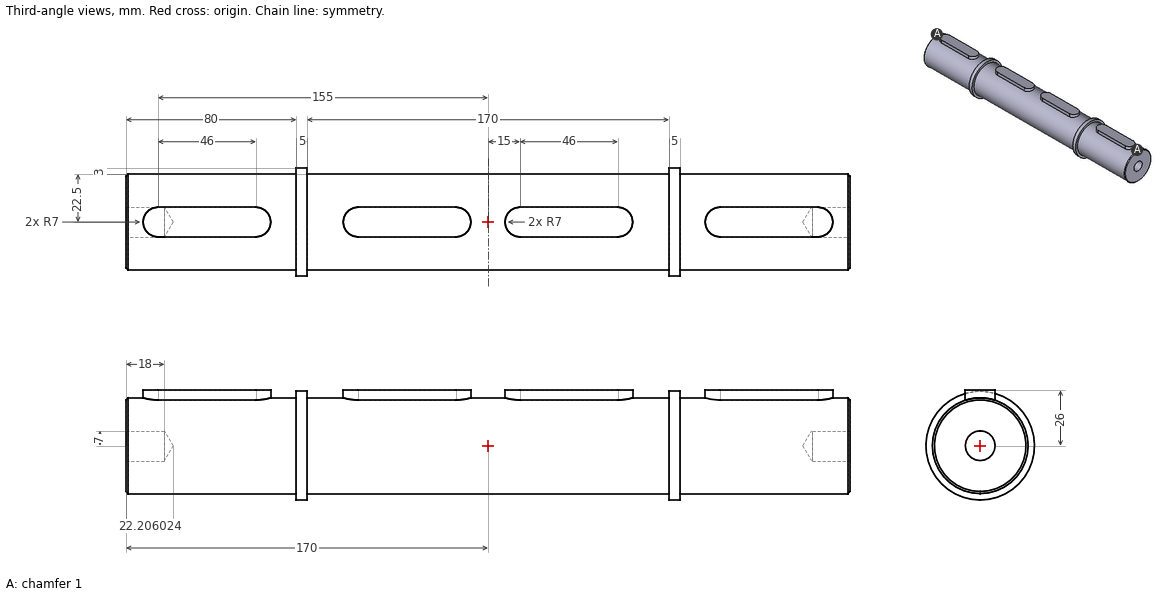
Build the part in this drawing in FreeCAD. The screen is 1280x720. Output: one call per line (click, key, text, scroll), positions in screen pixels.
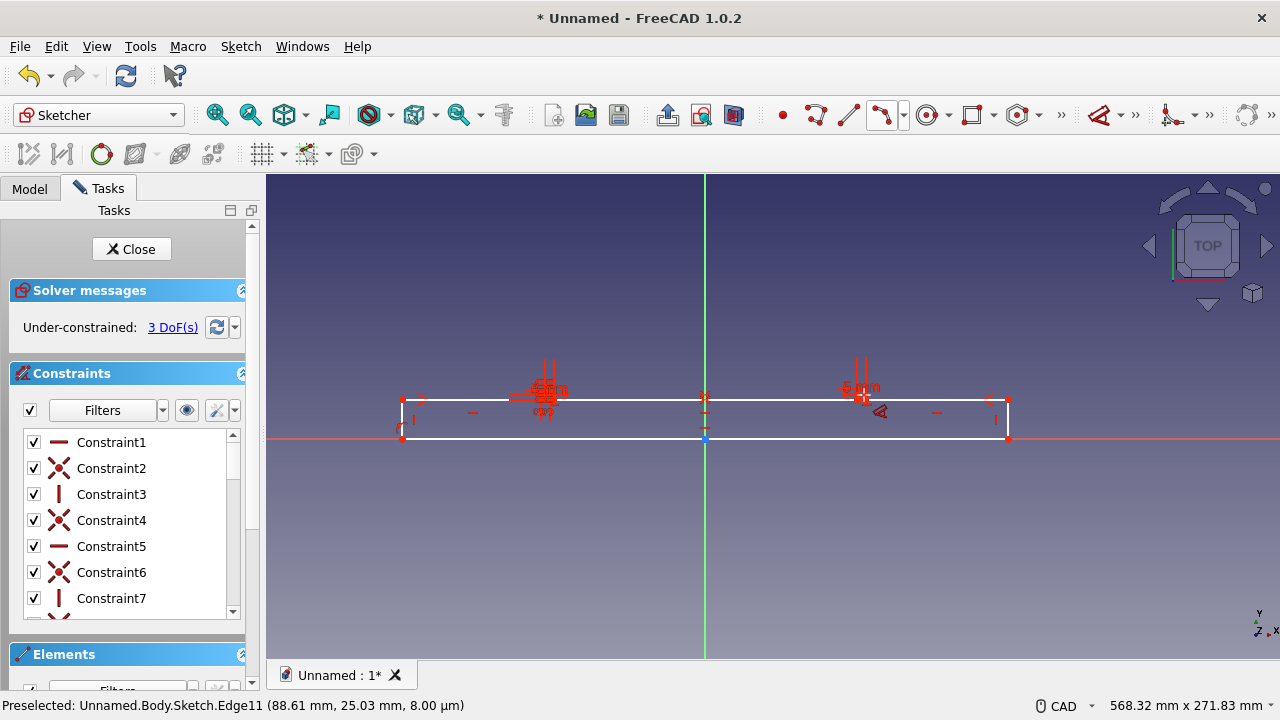
click(502, 400)
click(474, 366)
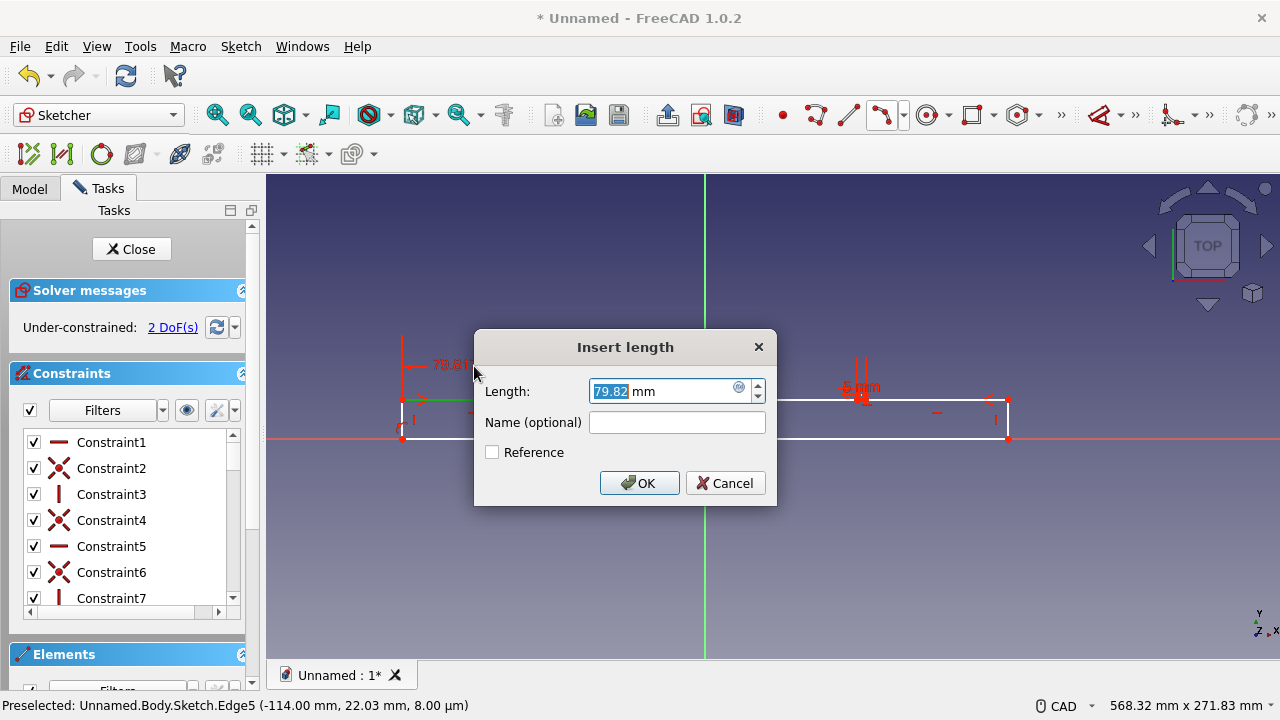
text(80)
key(Return)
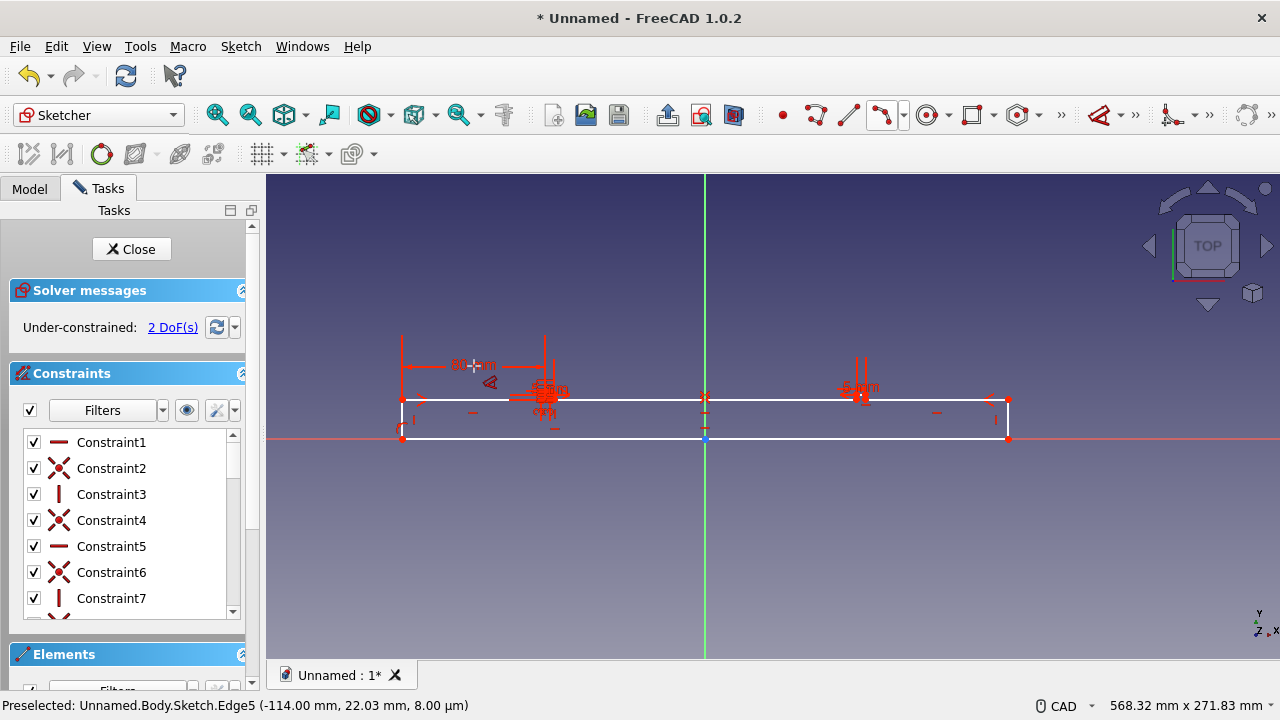
click(766, 400)
click(636, 366)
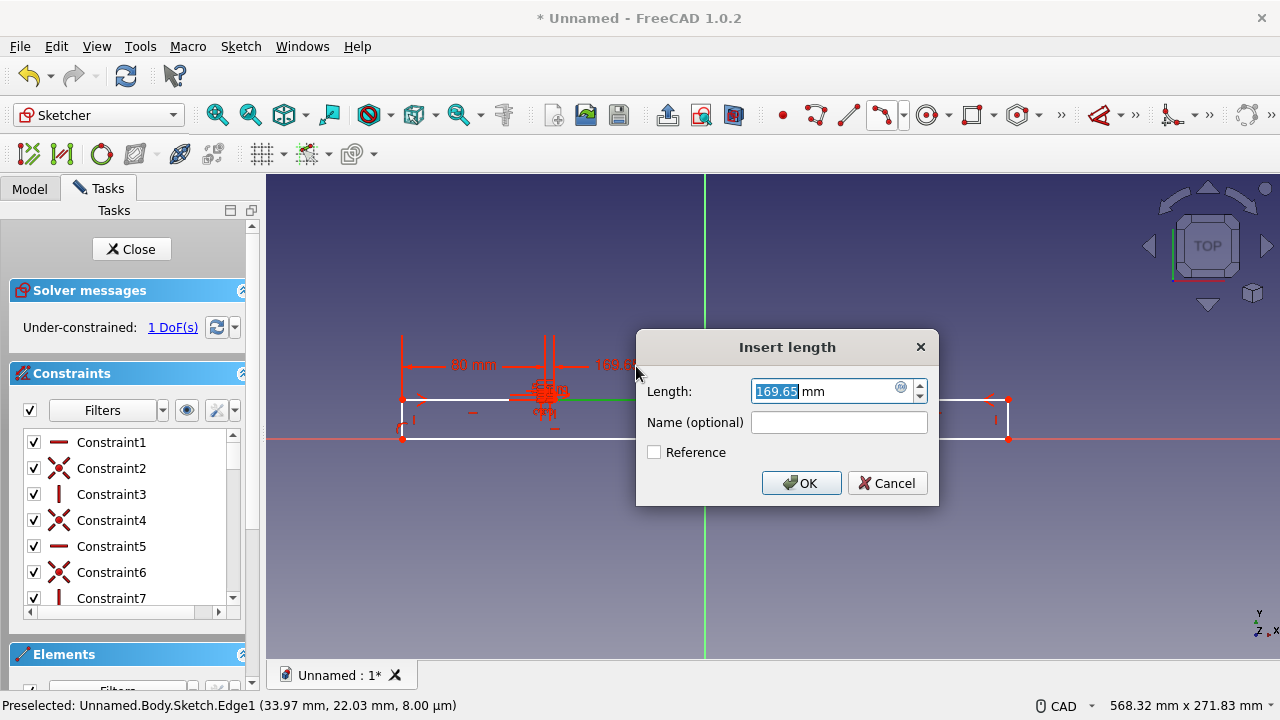
text(170)
key(Return)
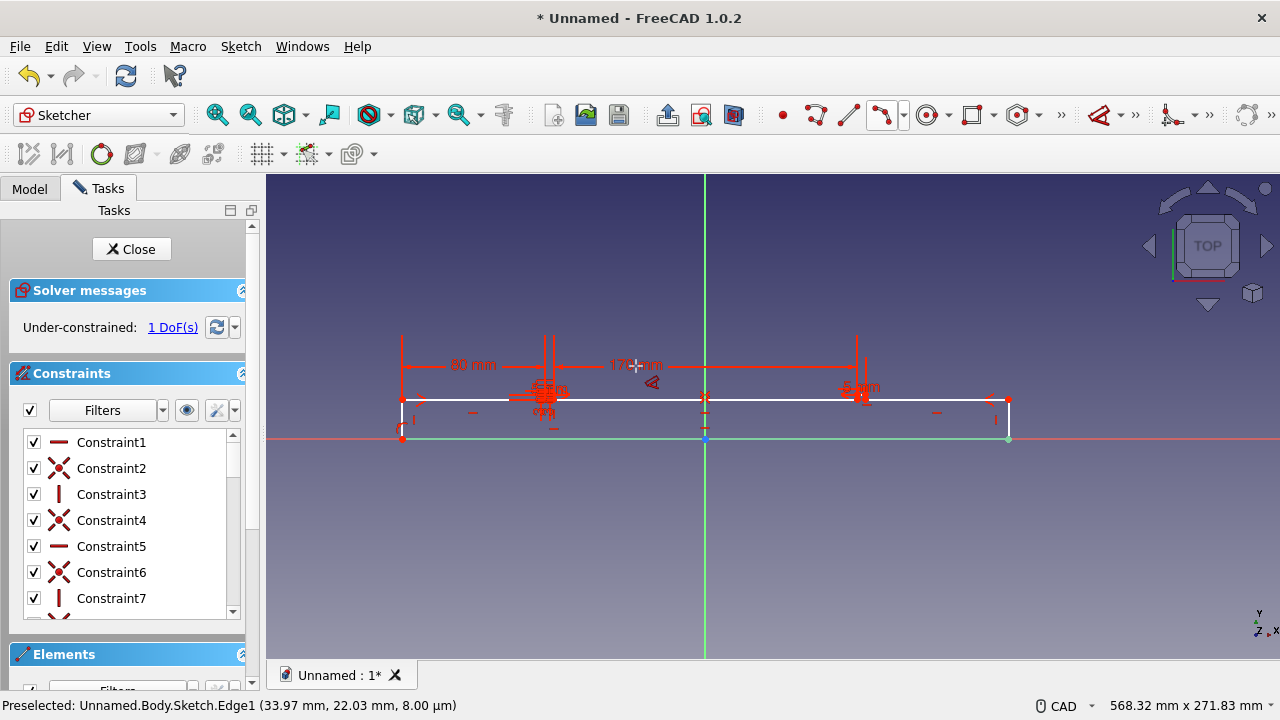
click(402, 412)
click(368, 420)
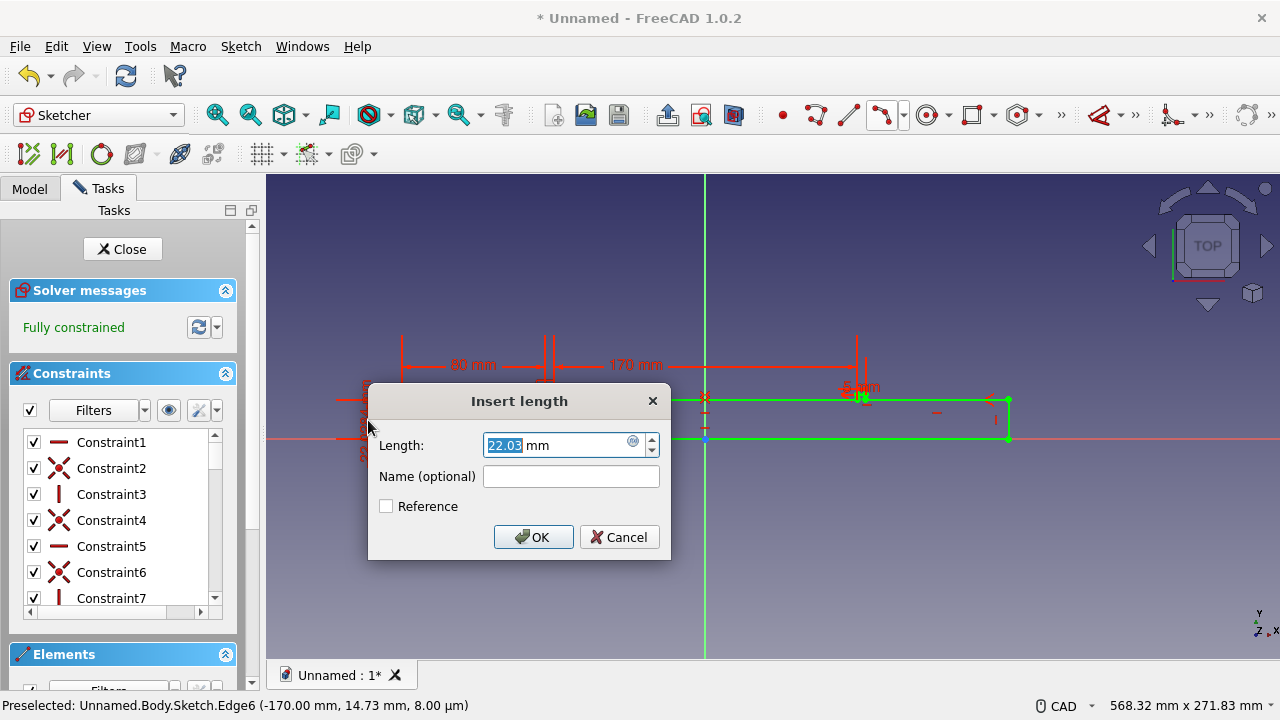
text(22.5)
key(Return)
key(Escape)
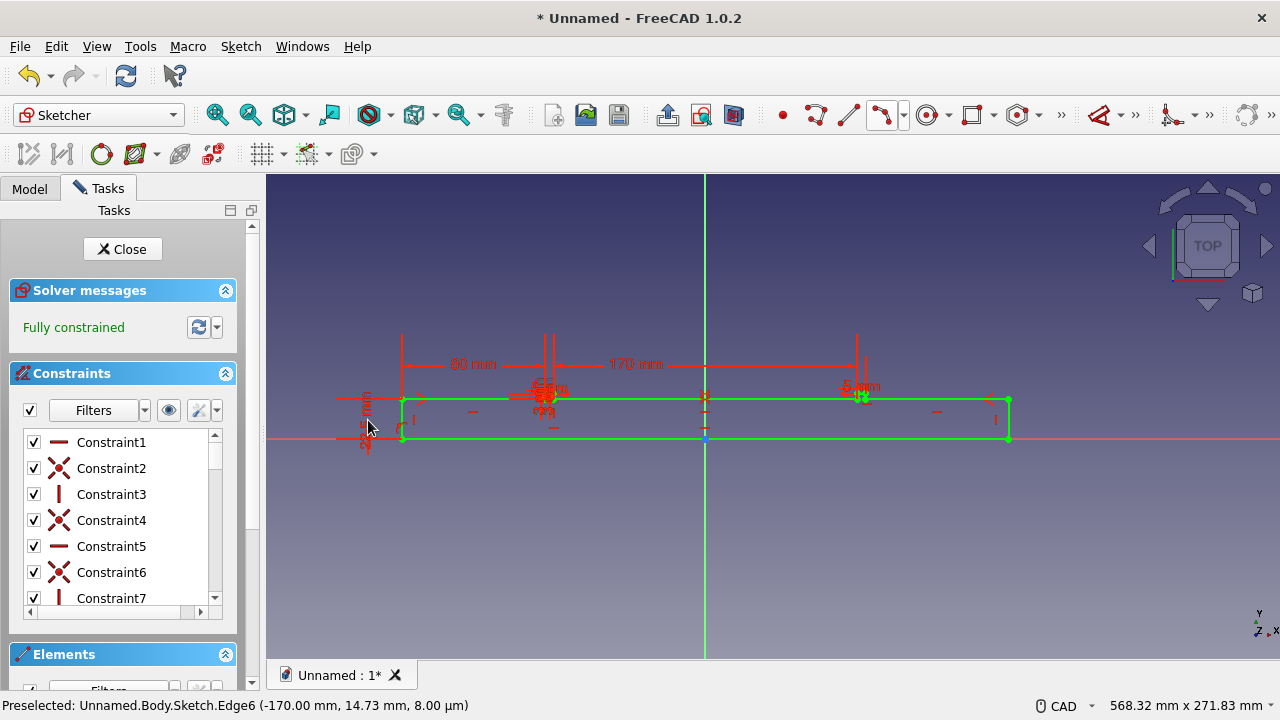
click(123, 249)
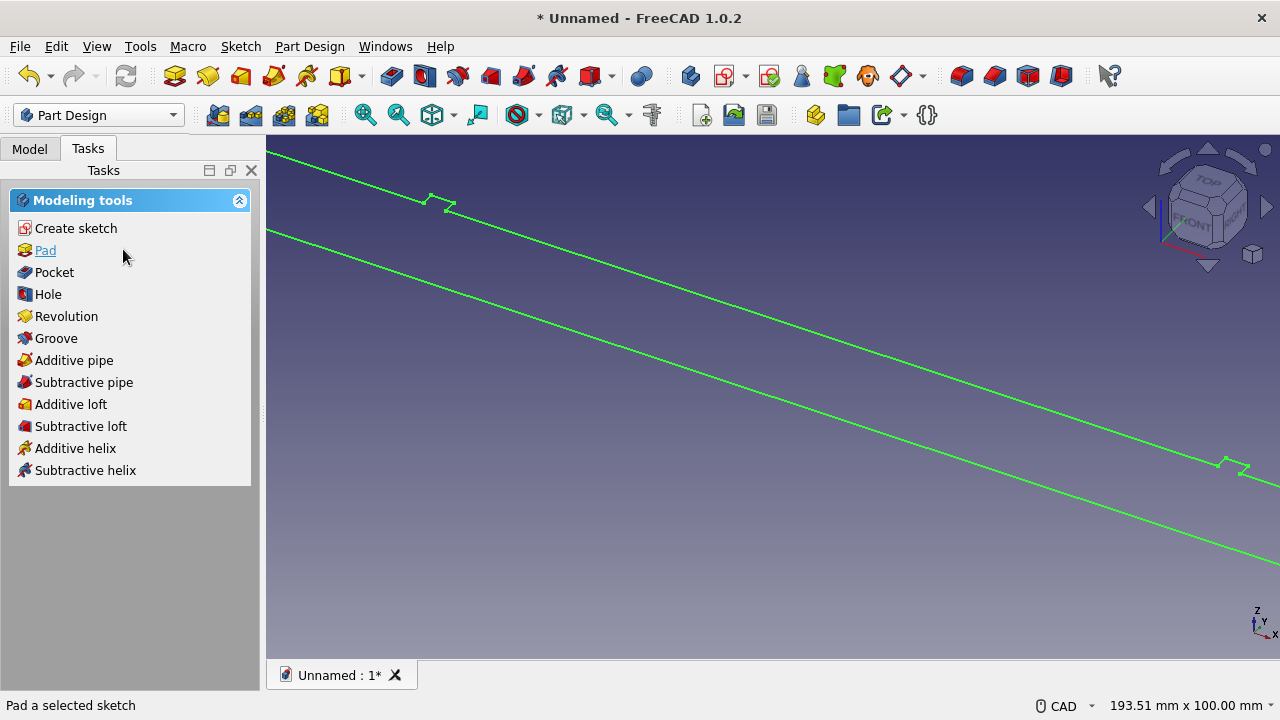
click(208, 76)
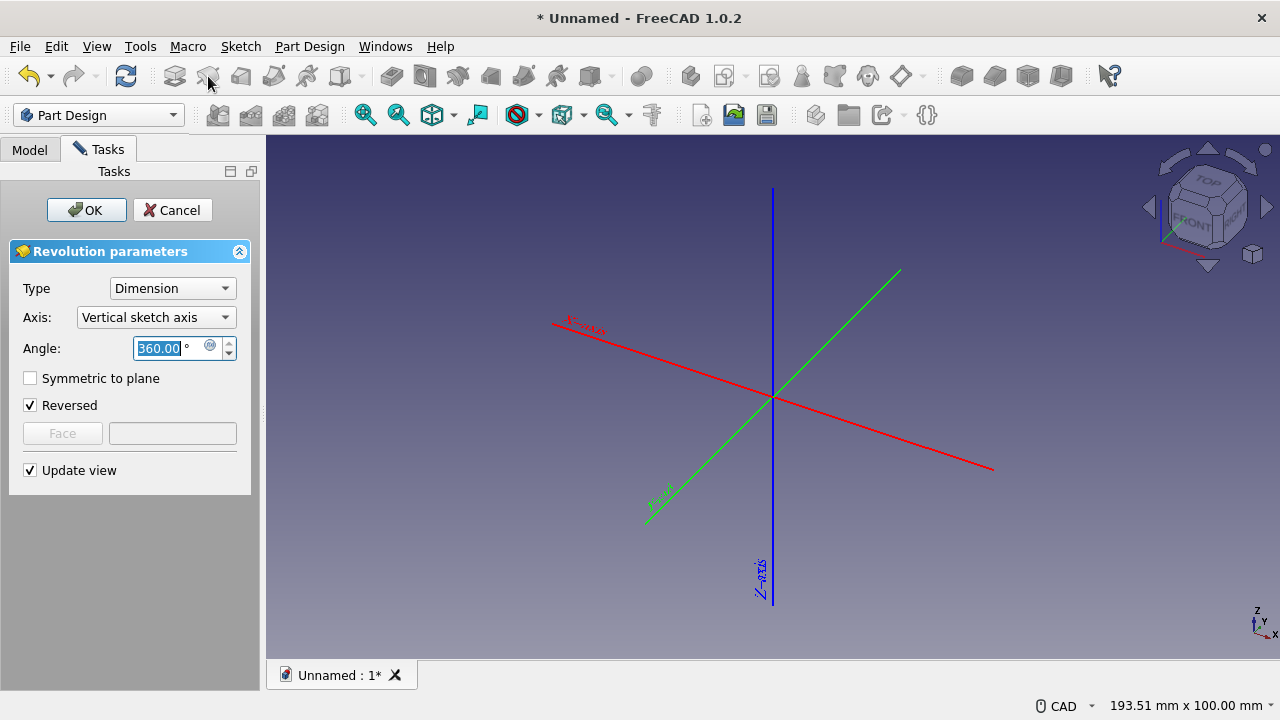
click(157, 318)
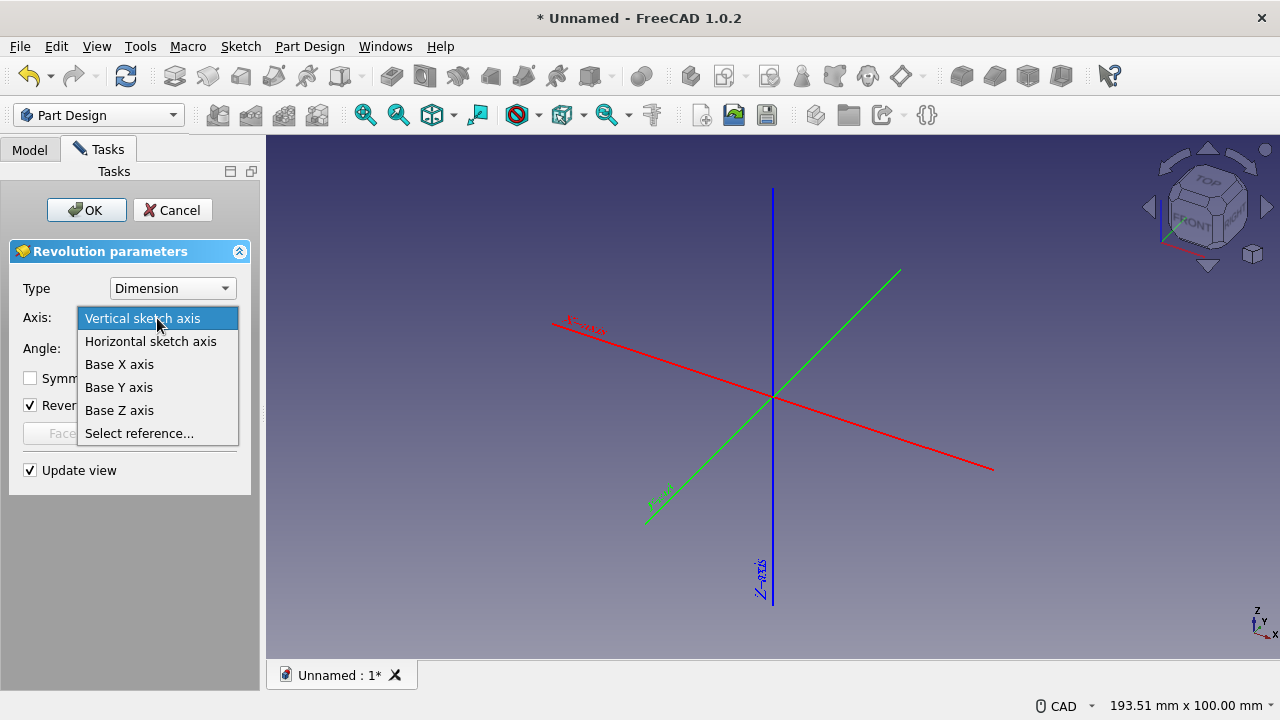
click(156, 342)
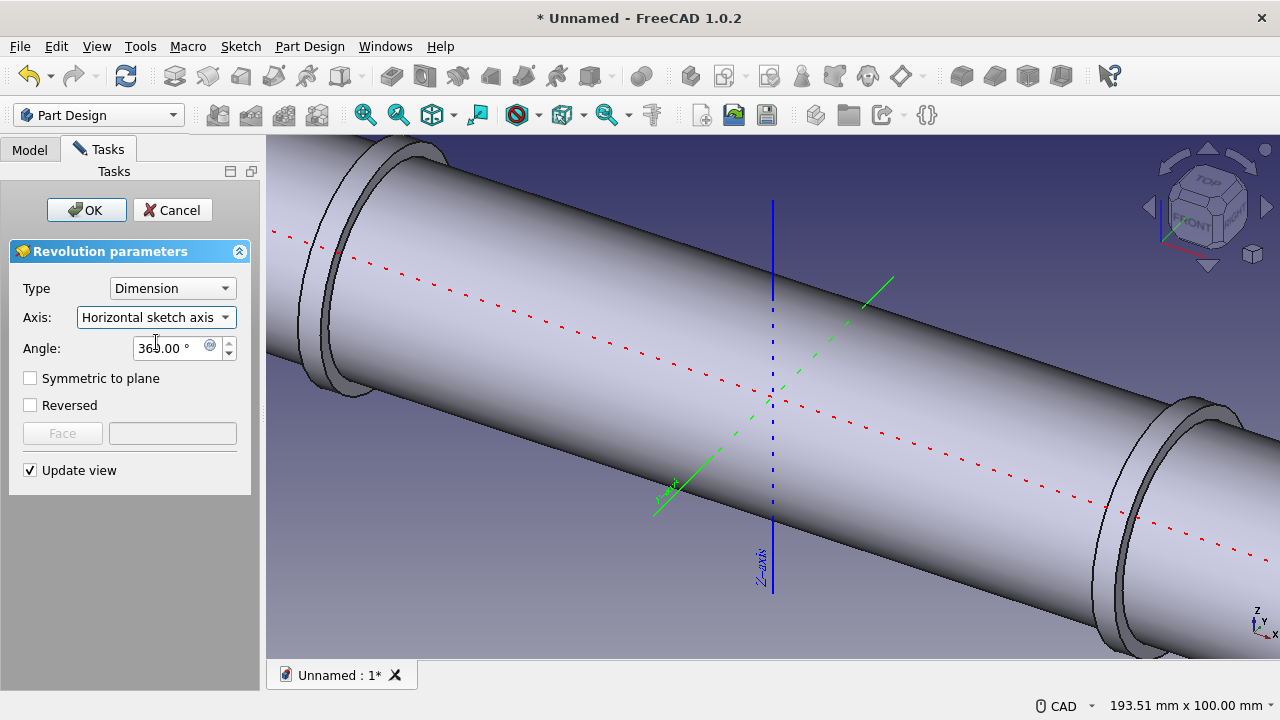
click(87, 210)